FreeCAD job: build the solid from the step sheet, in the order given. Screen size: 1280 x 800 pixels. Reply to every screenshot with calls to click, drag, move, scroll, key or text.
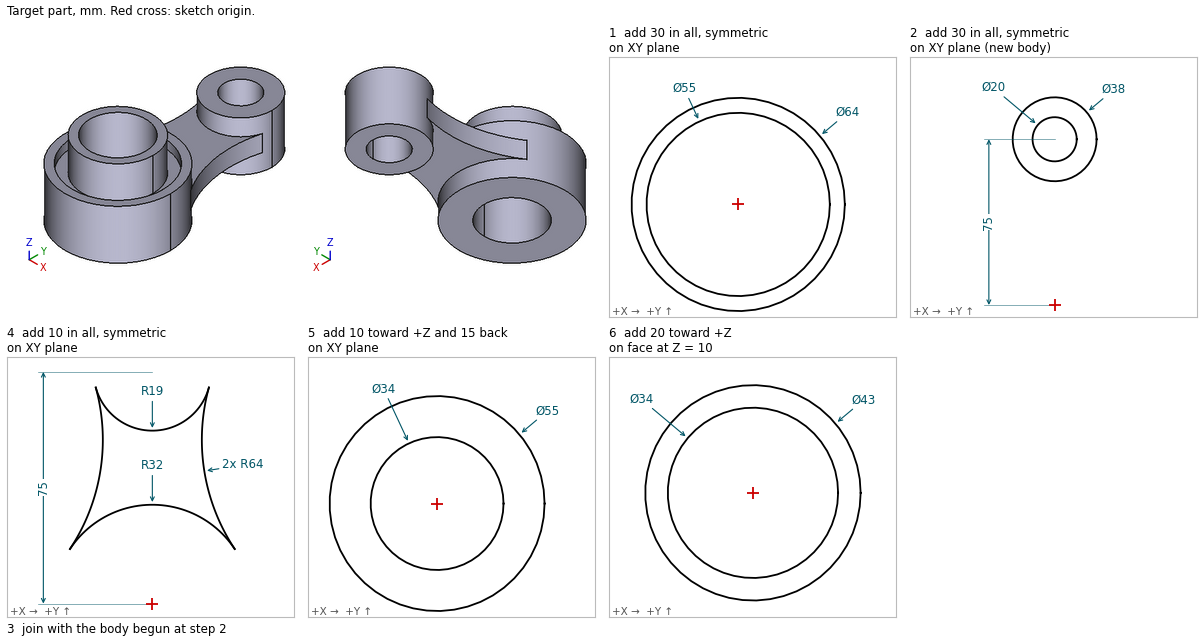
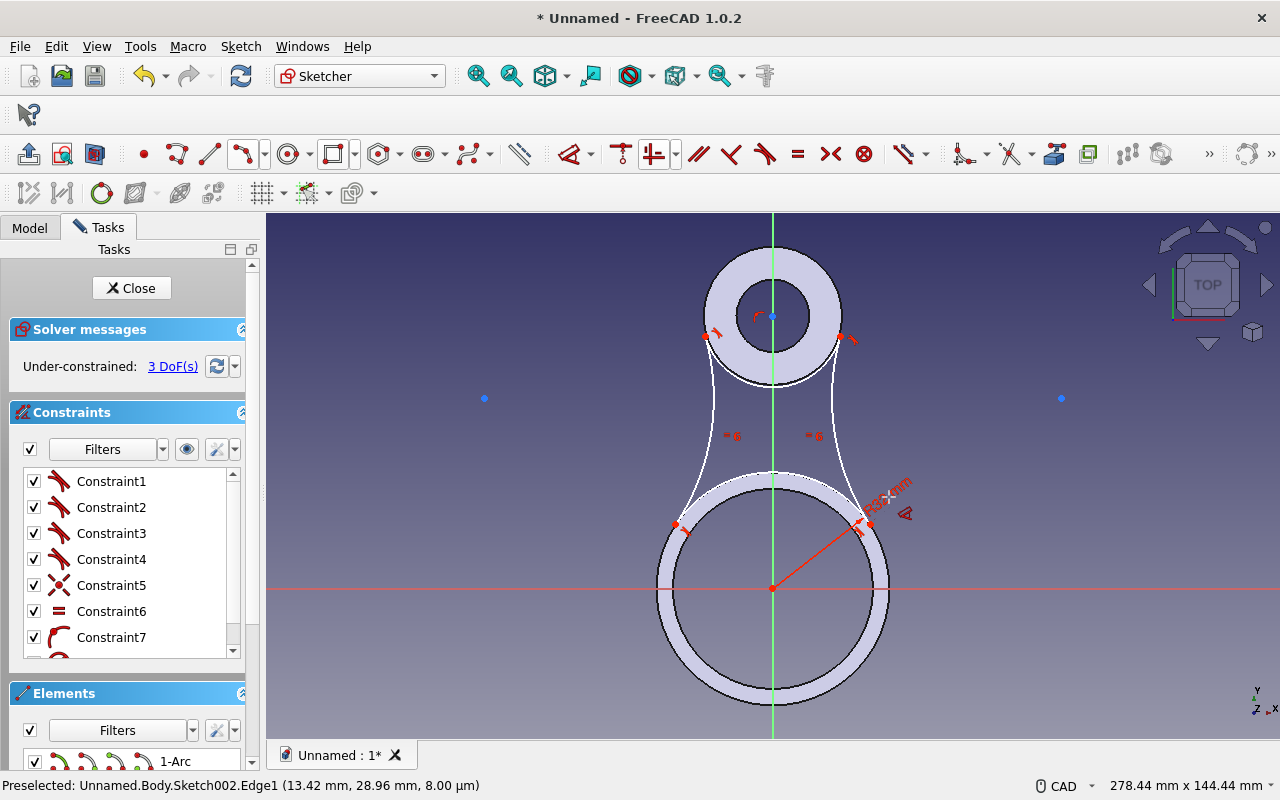
click(832, 394)
click(834, 269)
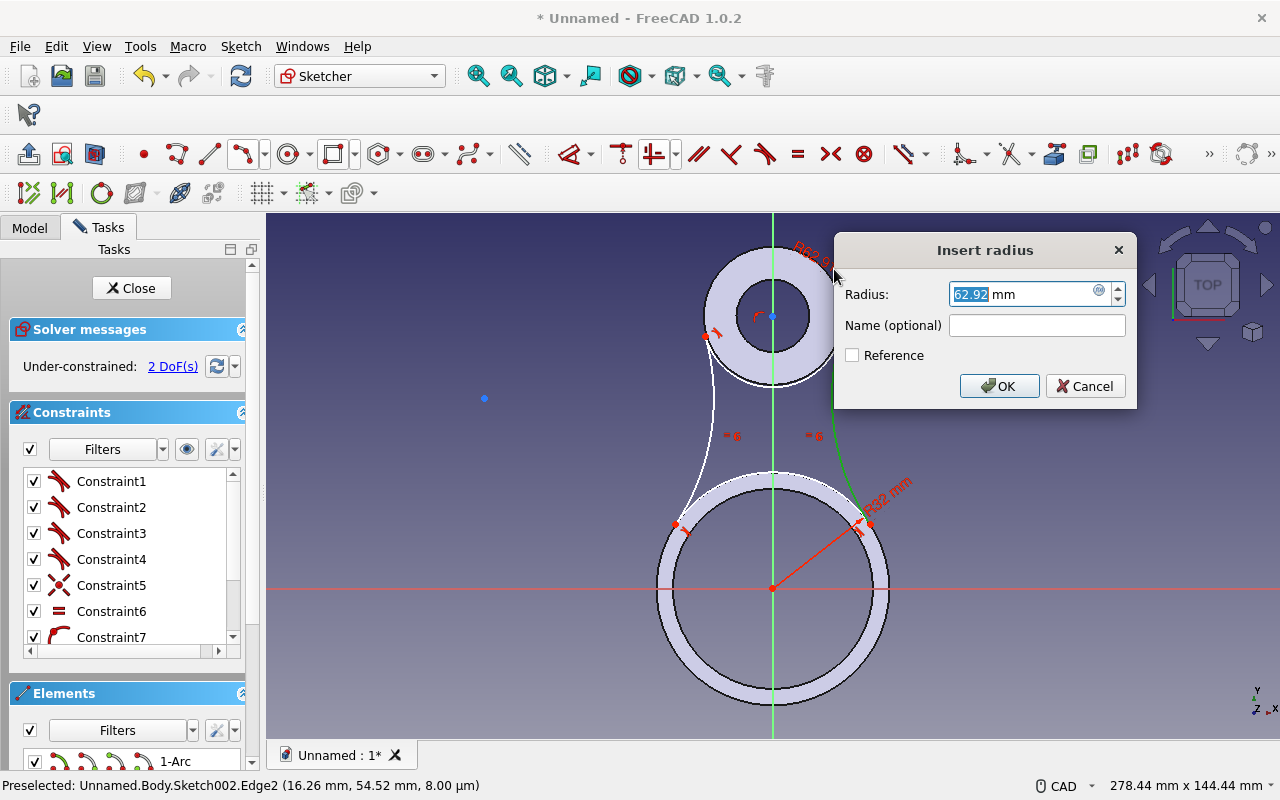
text(64)
key(Return)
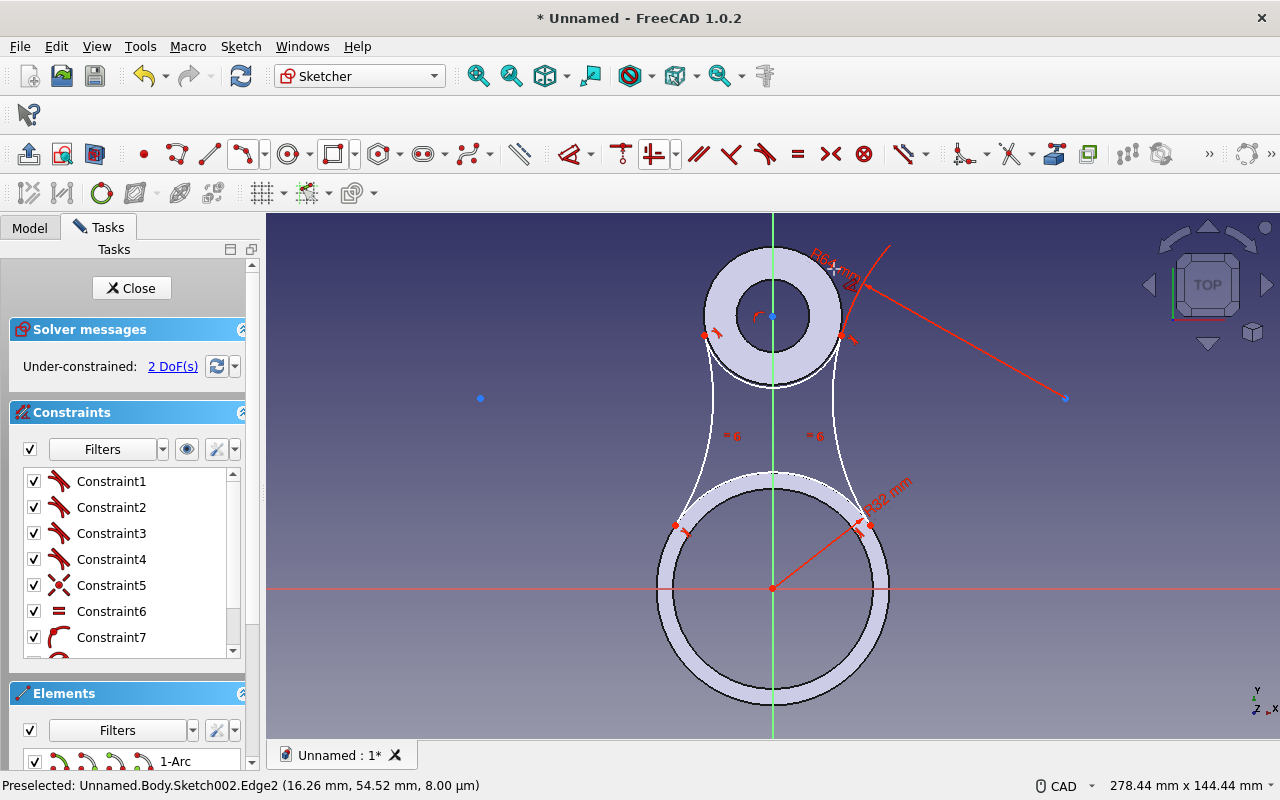
click(738, 378)
click(686, 371)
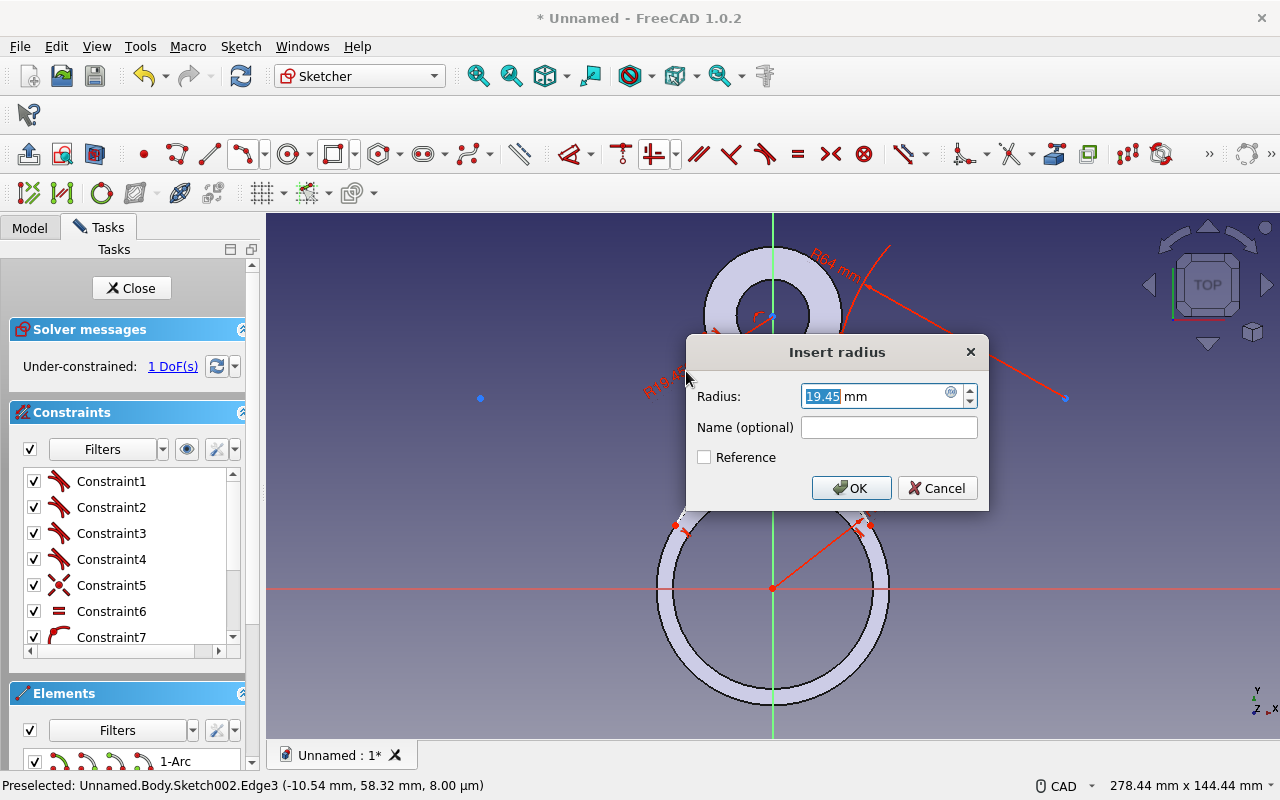
text(19)
key(Return)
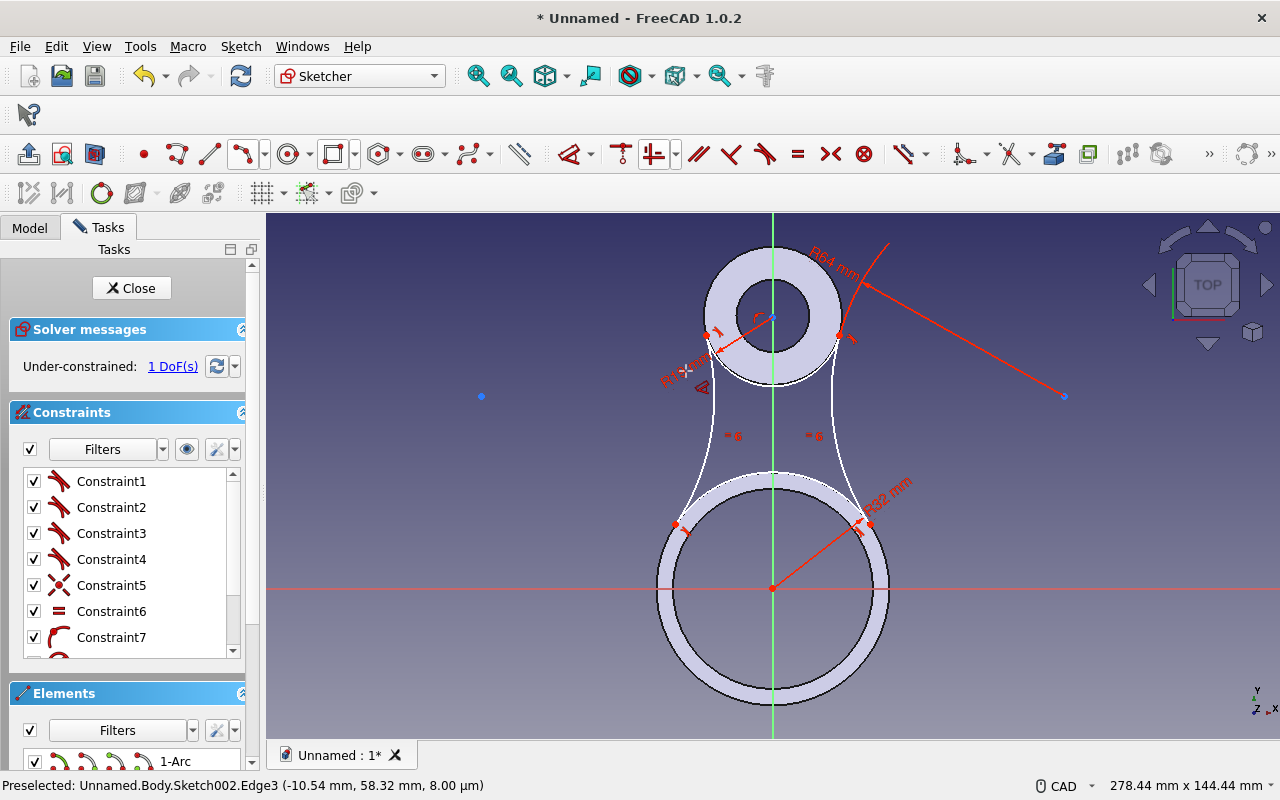
click(773, 317)
click(807, 453)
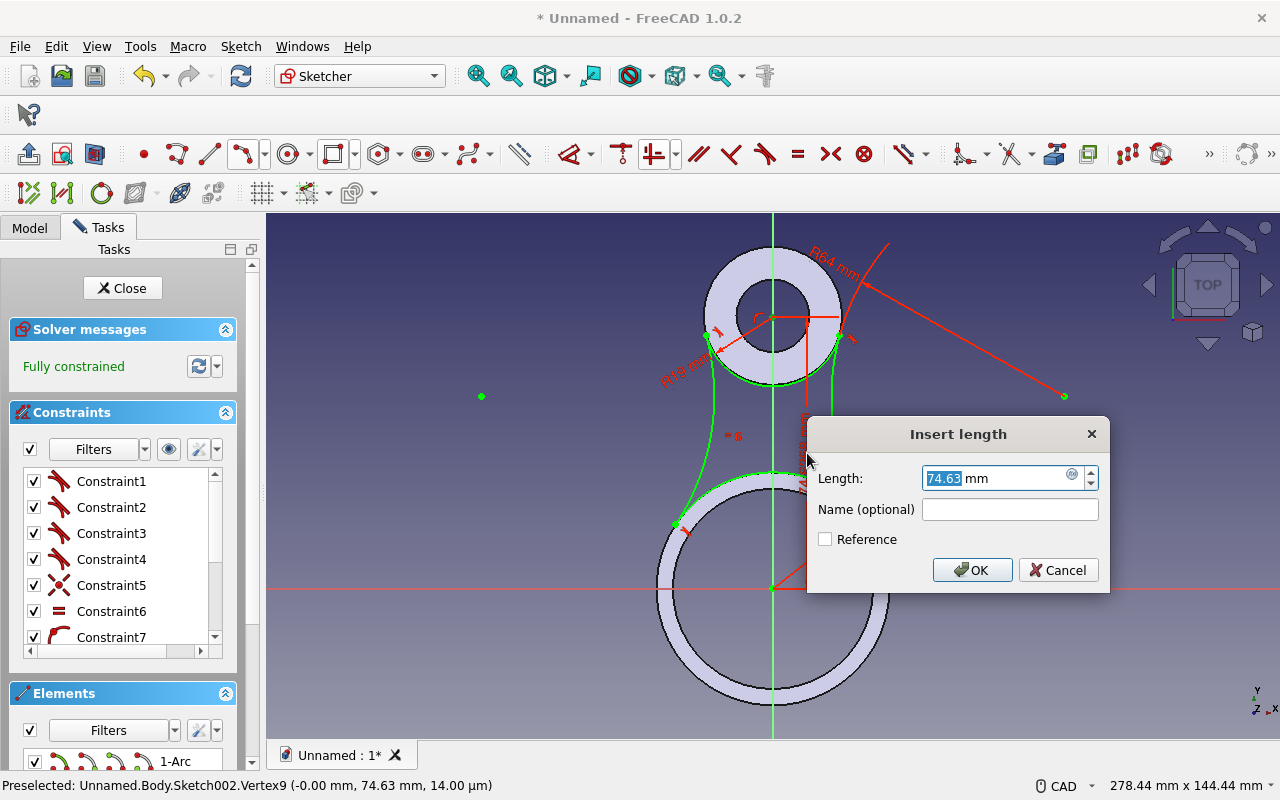
text(75)
key(Return)
key(Escape)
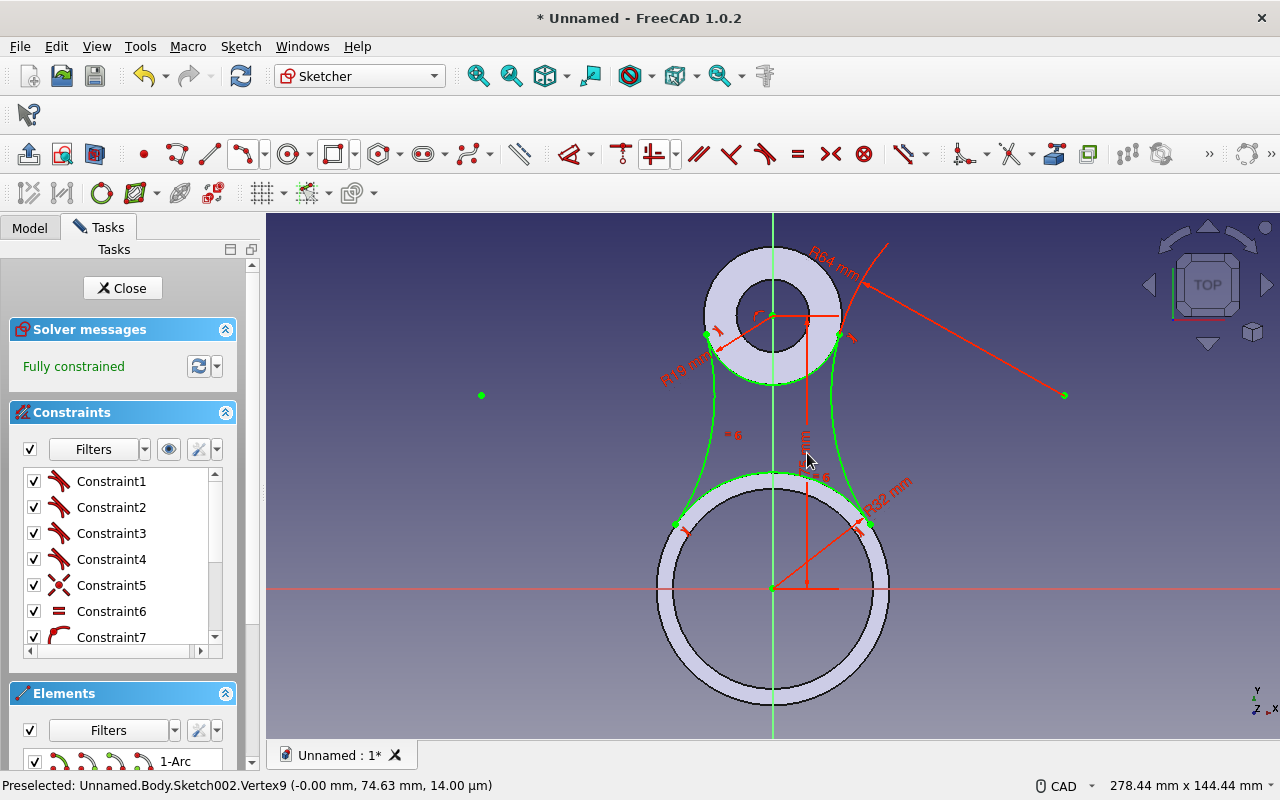
click(123, 288)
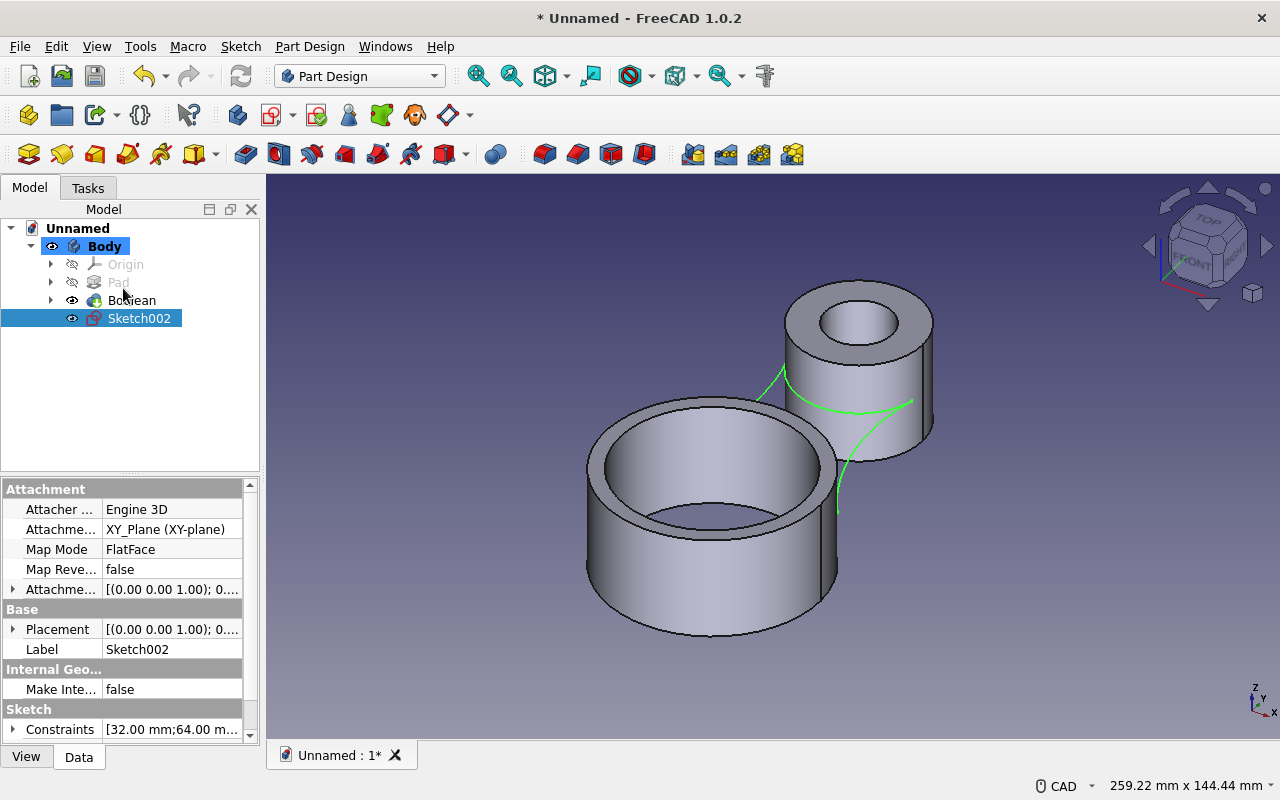
click(29, 154)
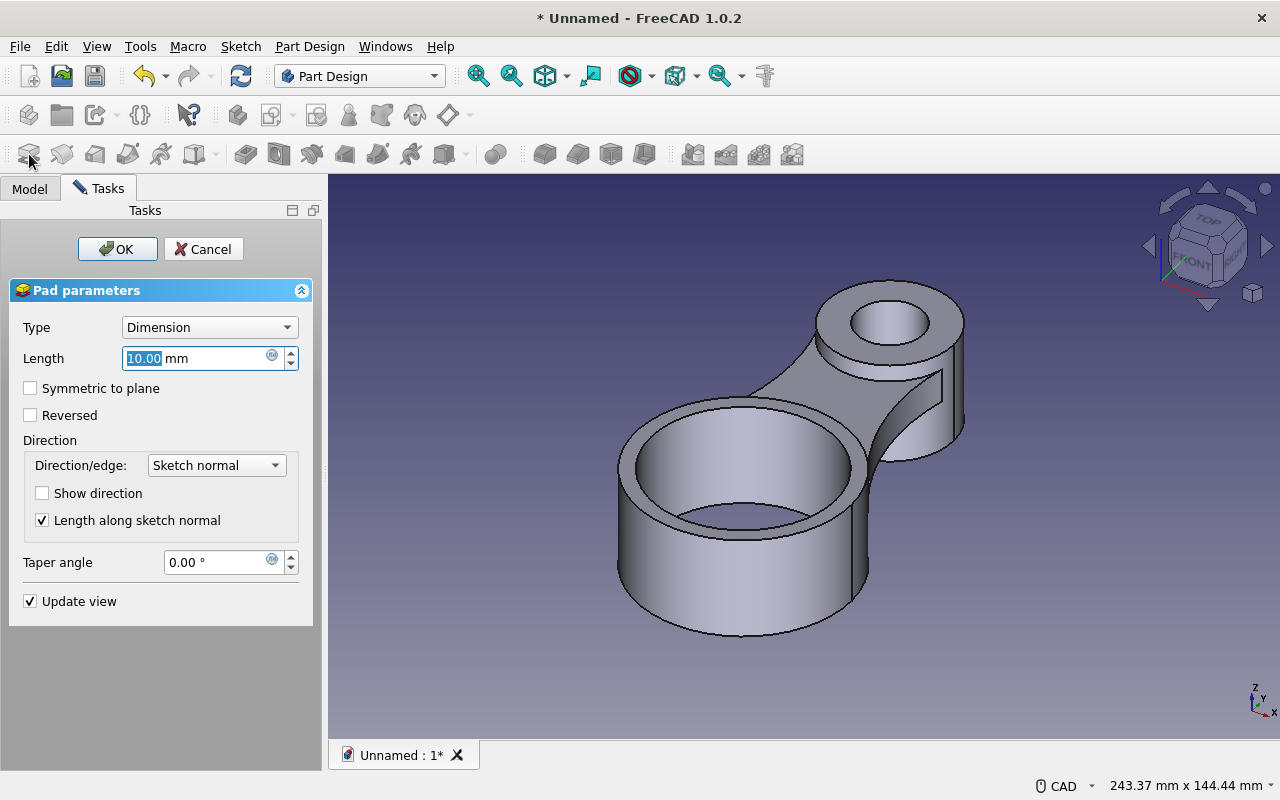
text(10)
key(Tab)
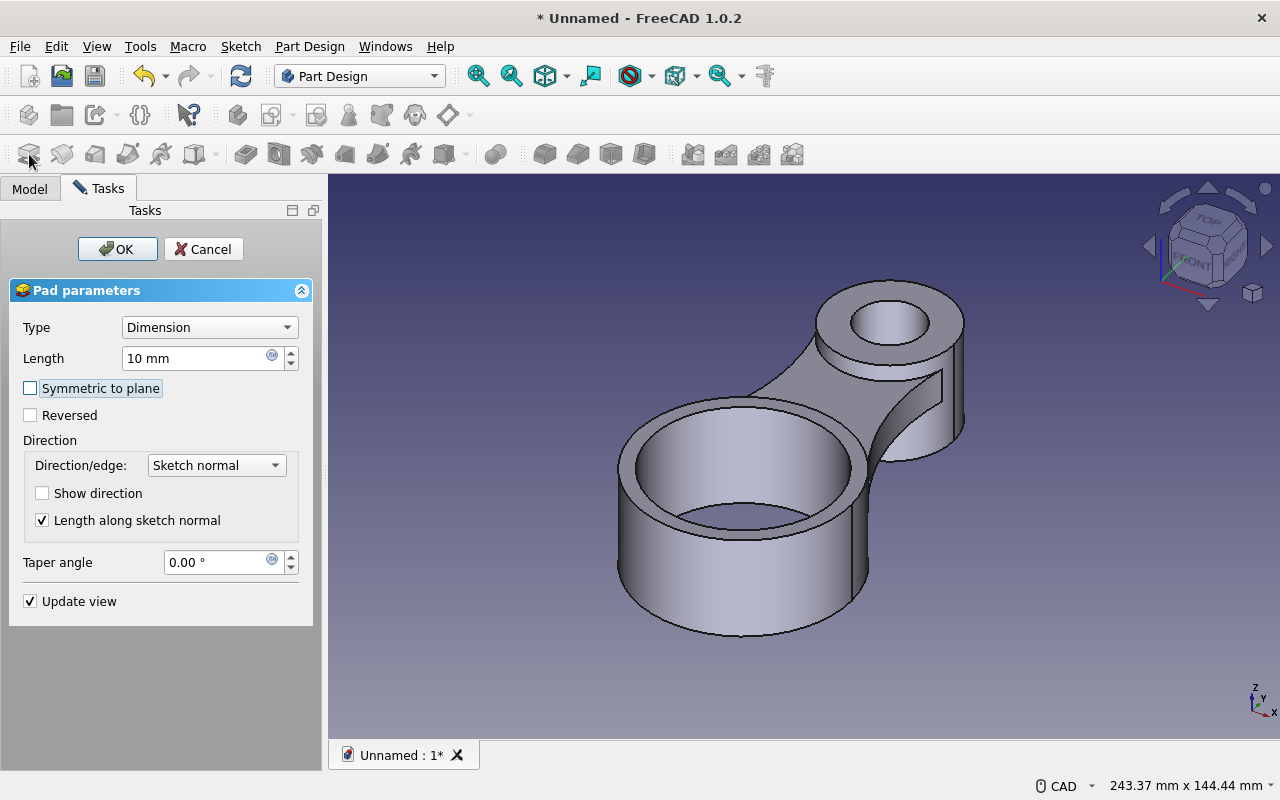
click(31, 388)